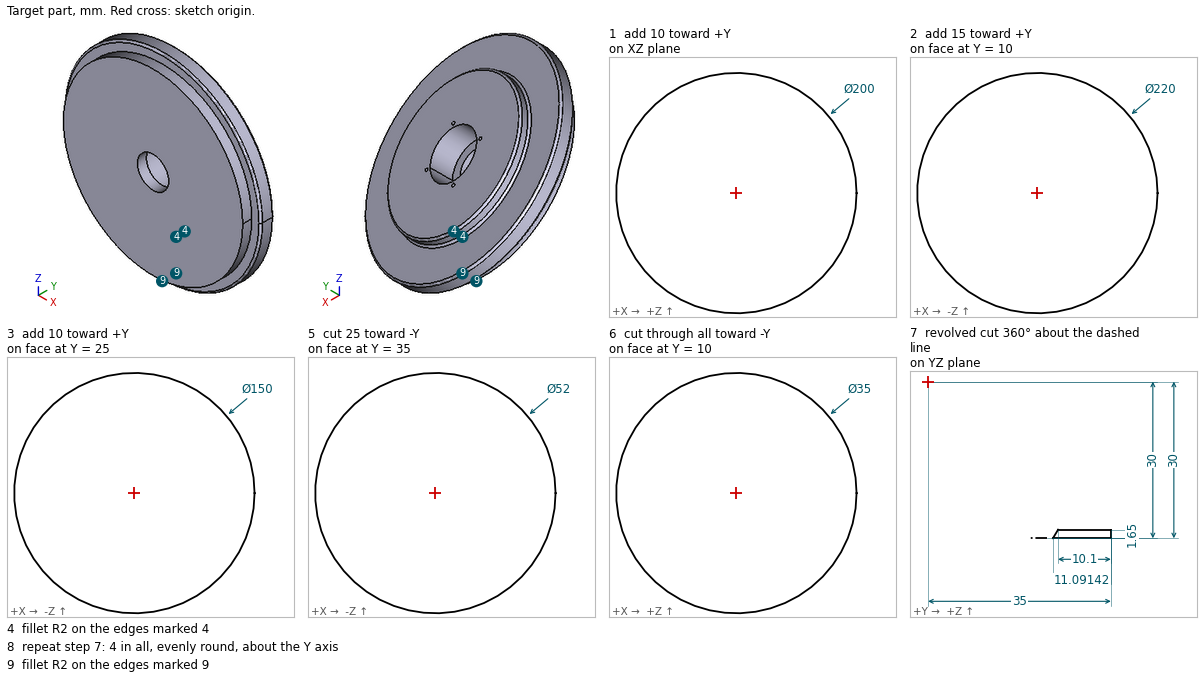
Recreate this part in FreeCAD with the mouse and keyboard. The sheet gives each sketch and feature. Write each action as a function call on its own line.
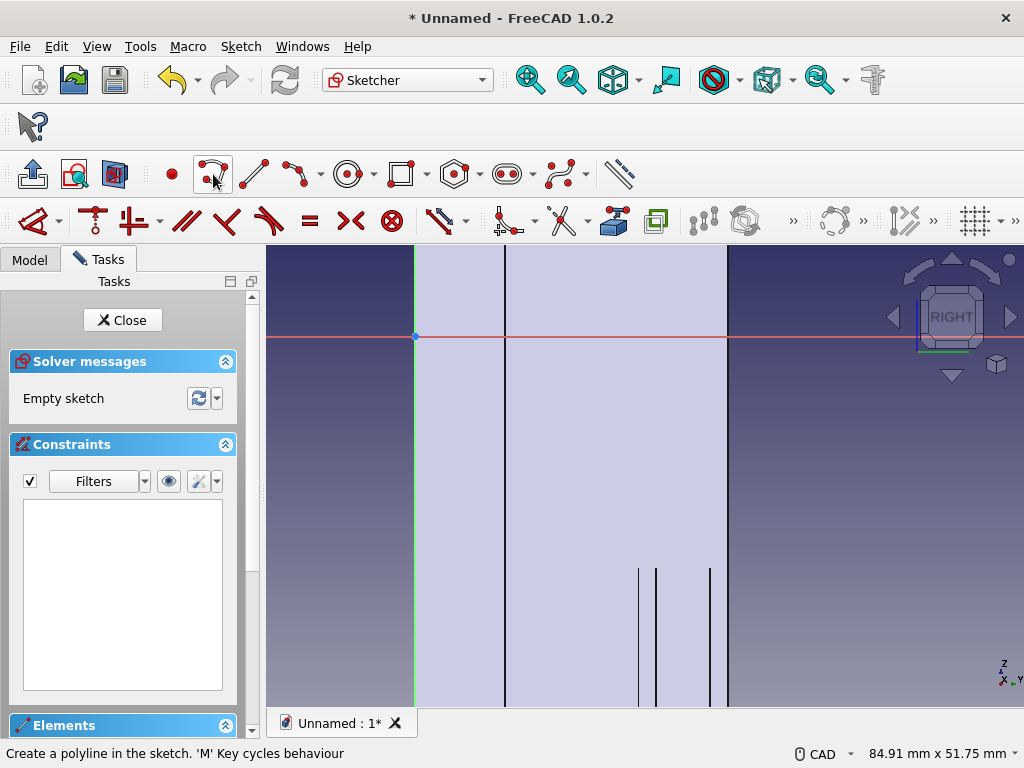
click(638, 590)
click(629, 605)
click(728, 605)
click(728, 590)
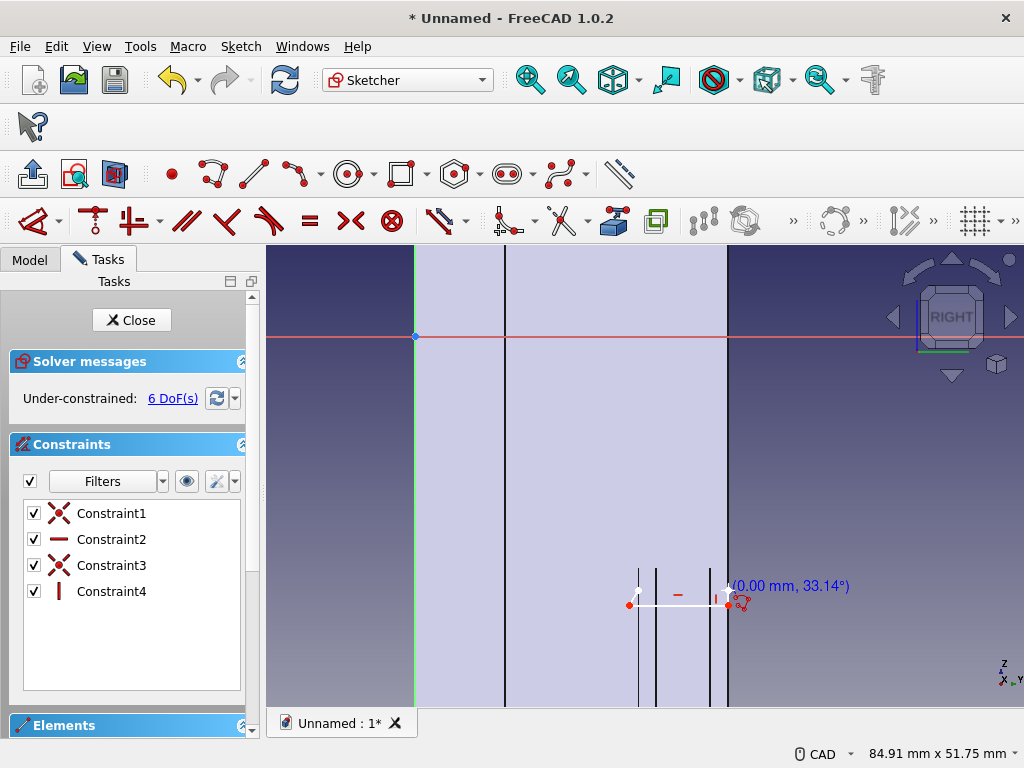
scroll(638, 590, up, 4)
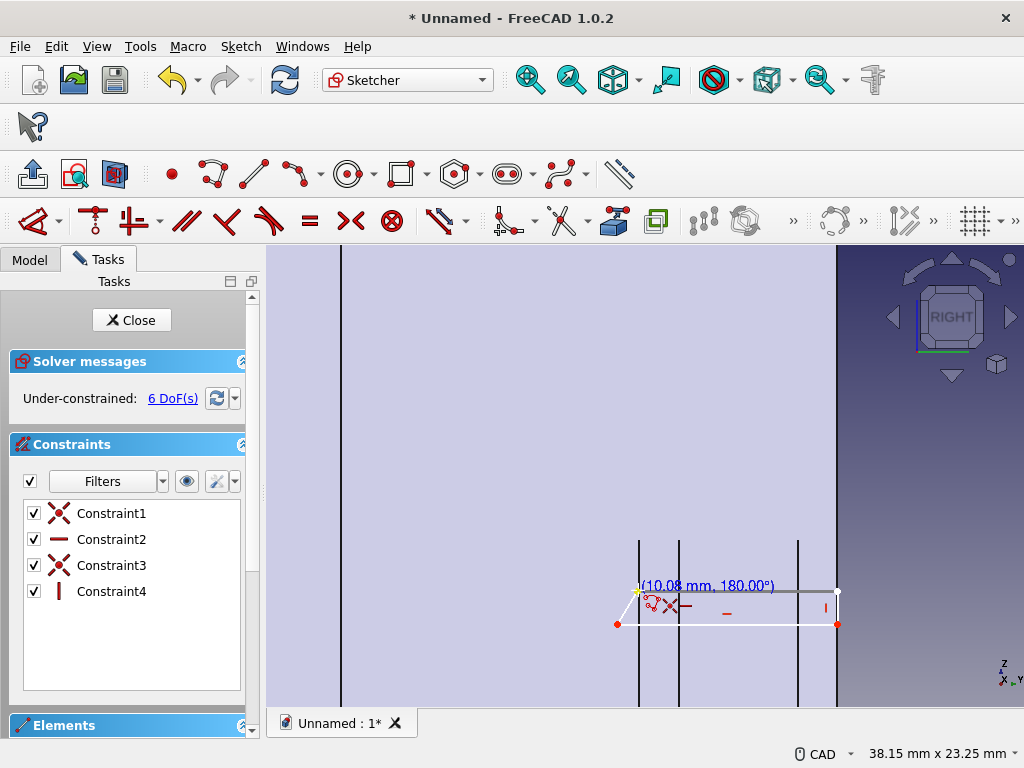
click(637, 591)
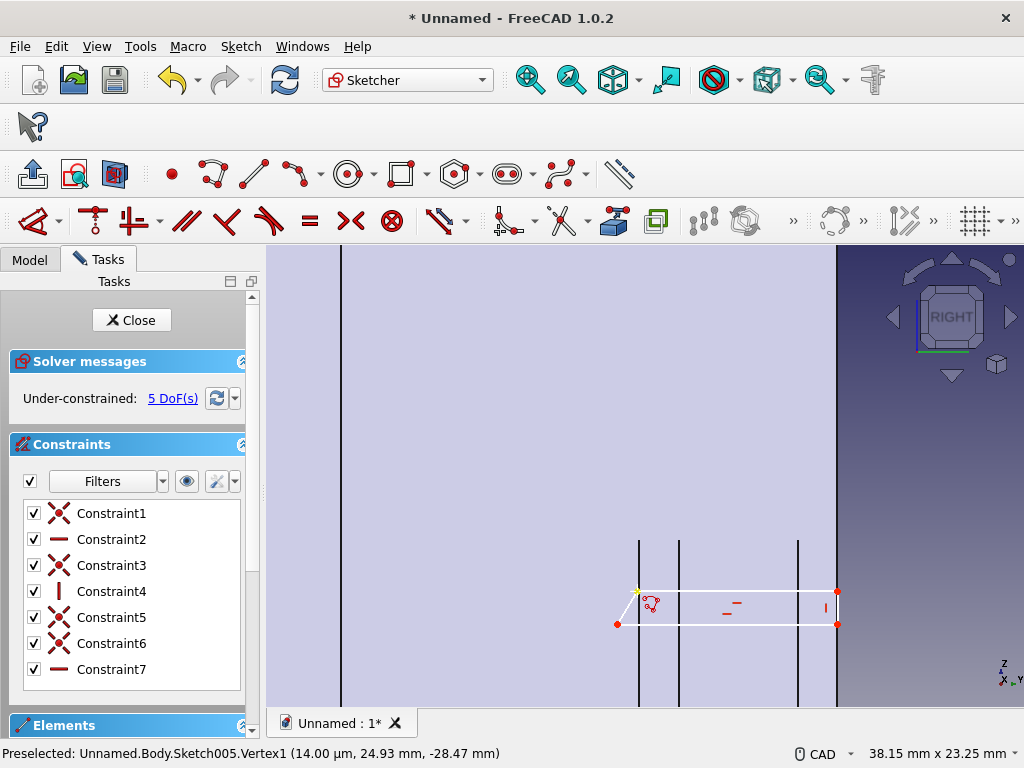
click(254, 174)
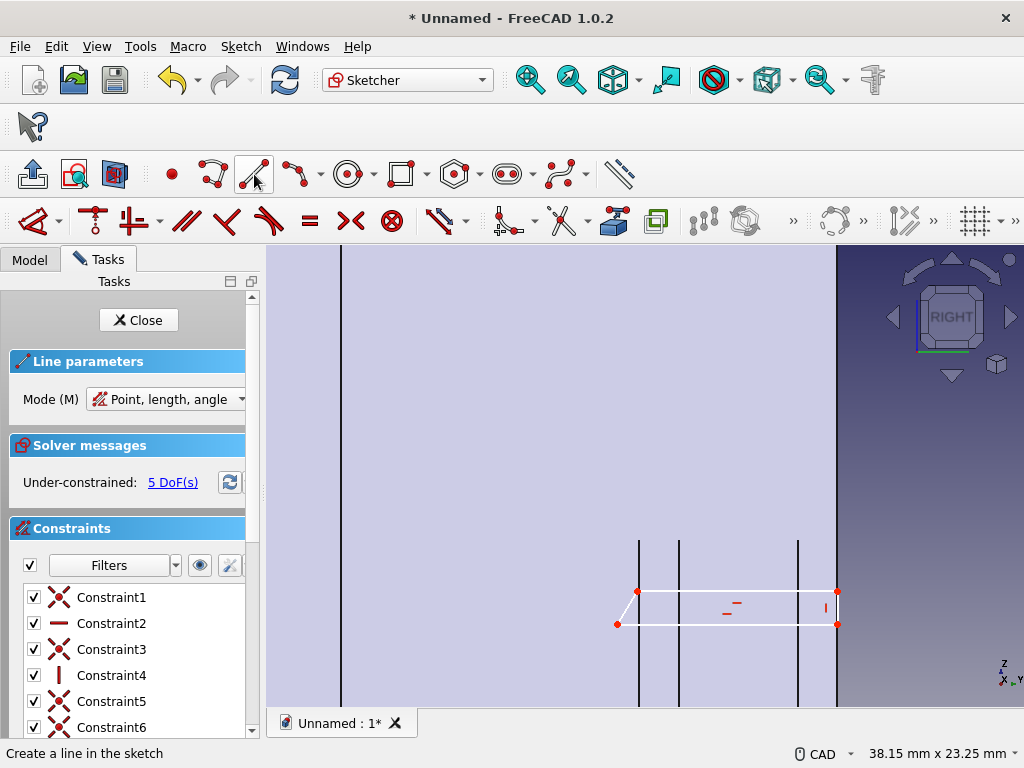
click(595, 622)
click(529, 622)
key(Escape)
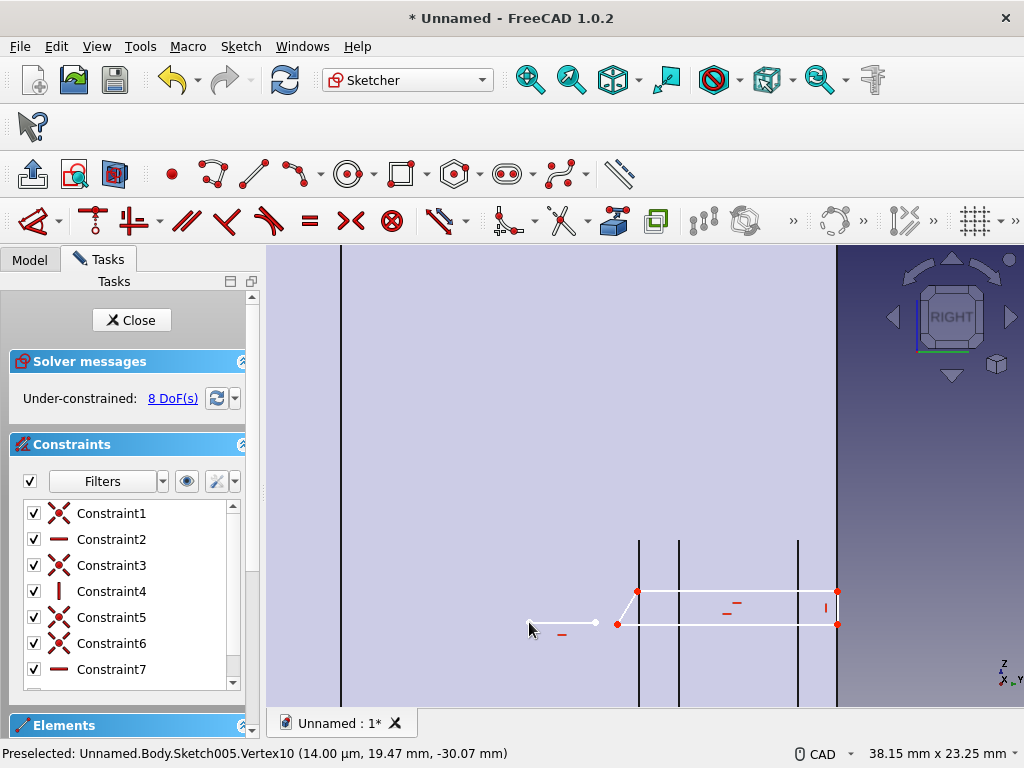
click(575, 623)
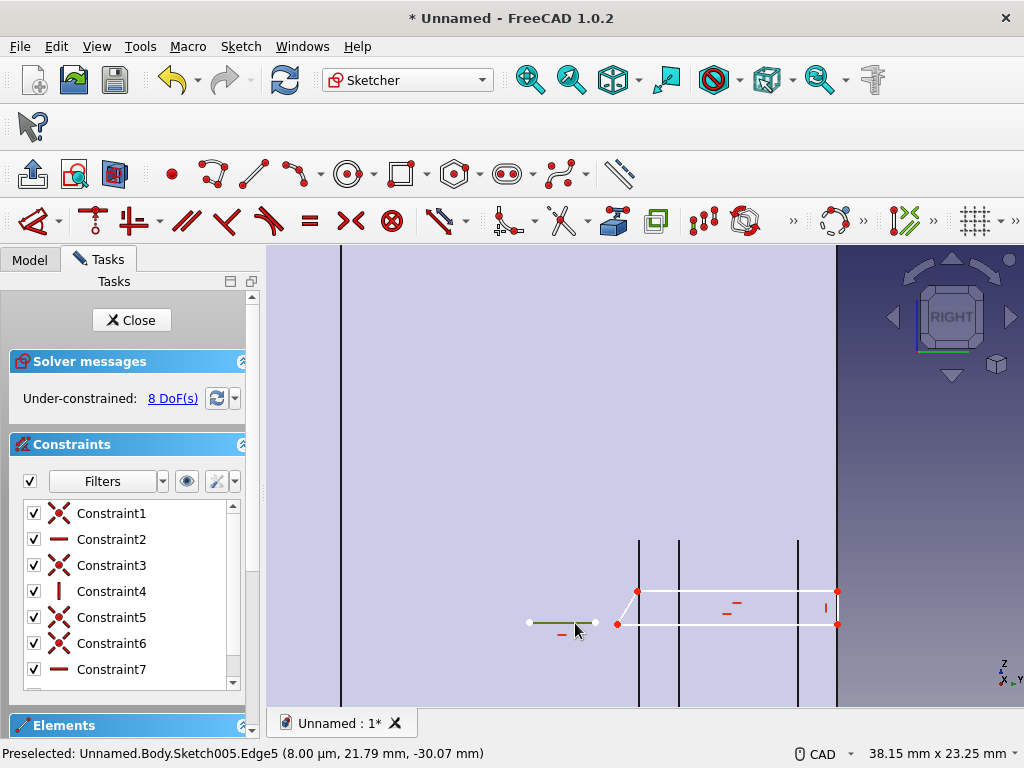
click(620, 174)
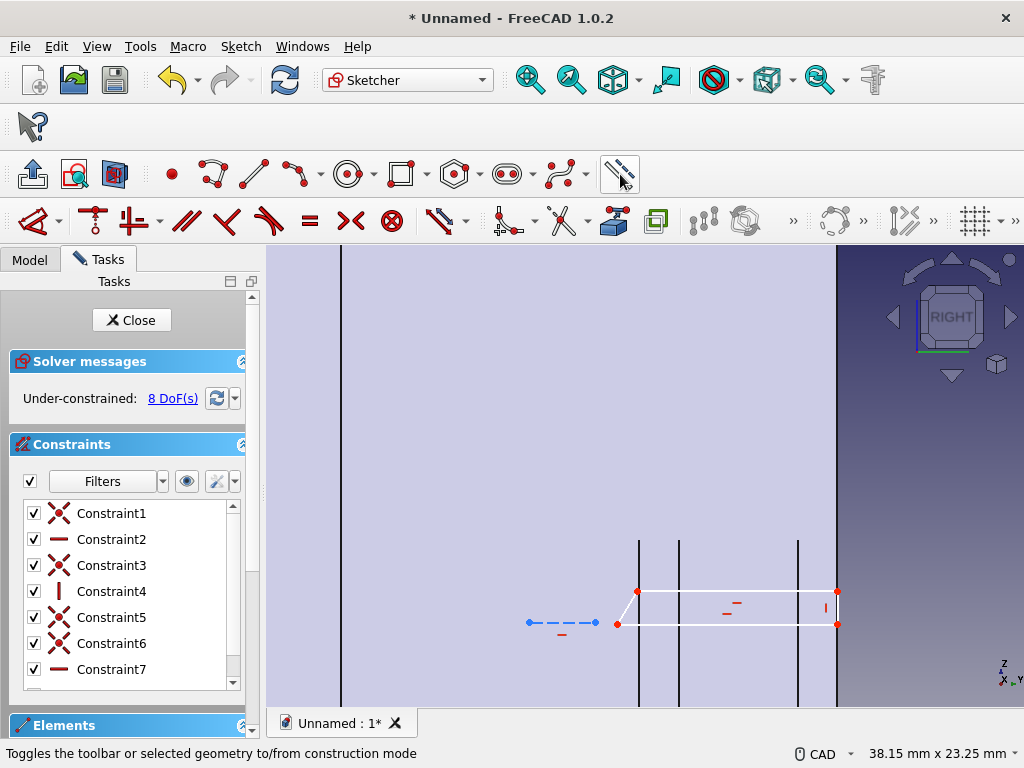
click(32, 222)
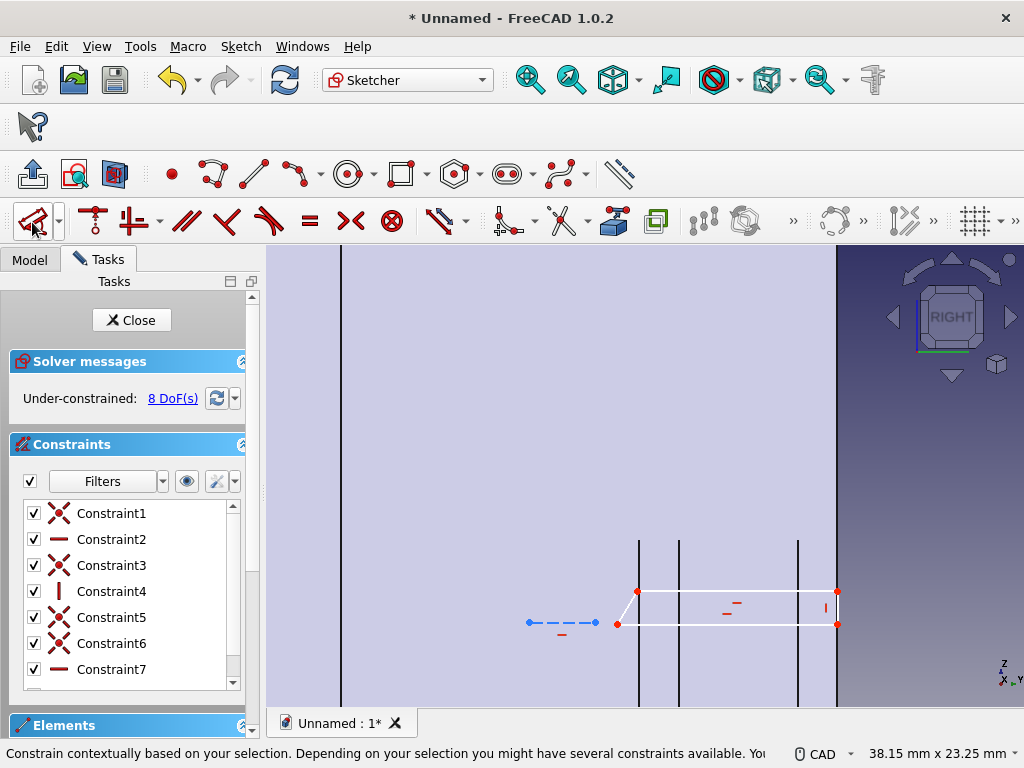
click(617, 625)
click(651, 449)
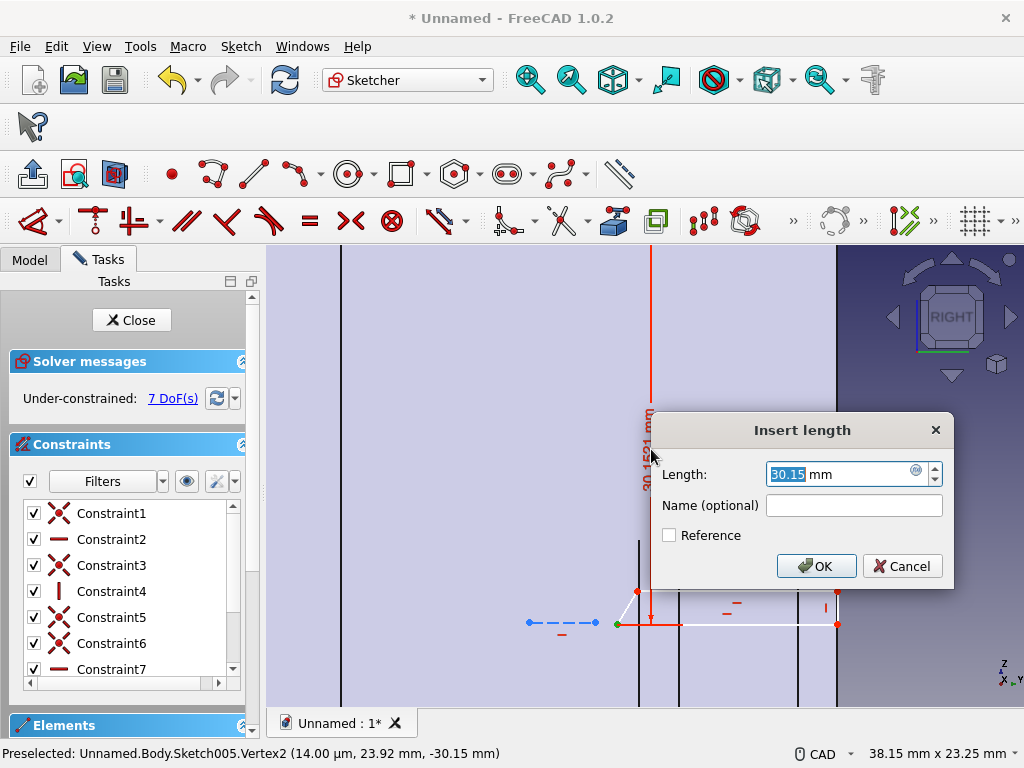
text(30)
key(Return)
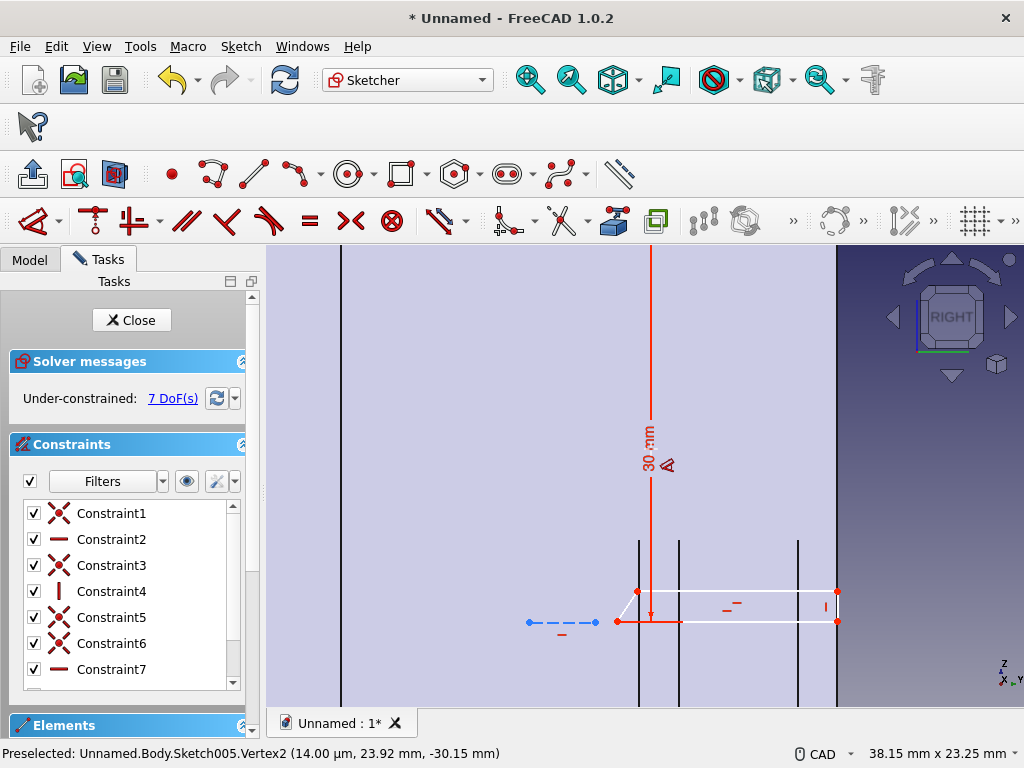
click(838, 622)
click(566, 656)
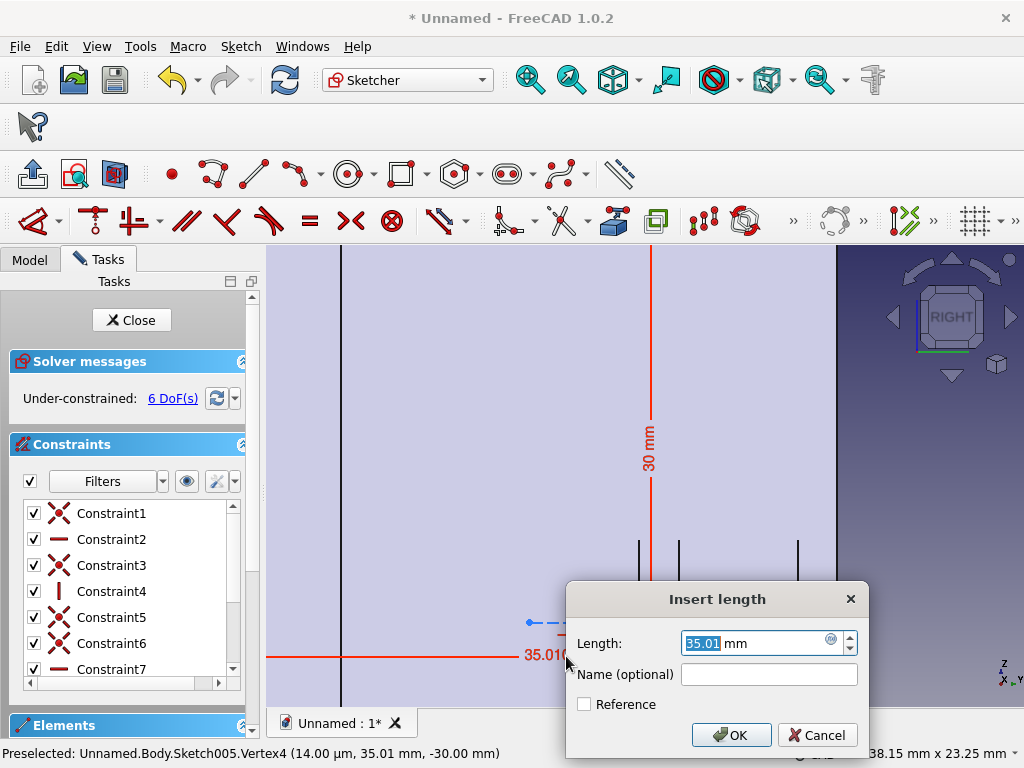
text(35)
key(Return)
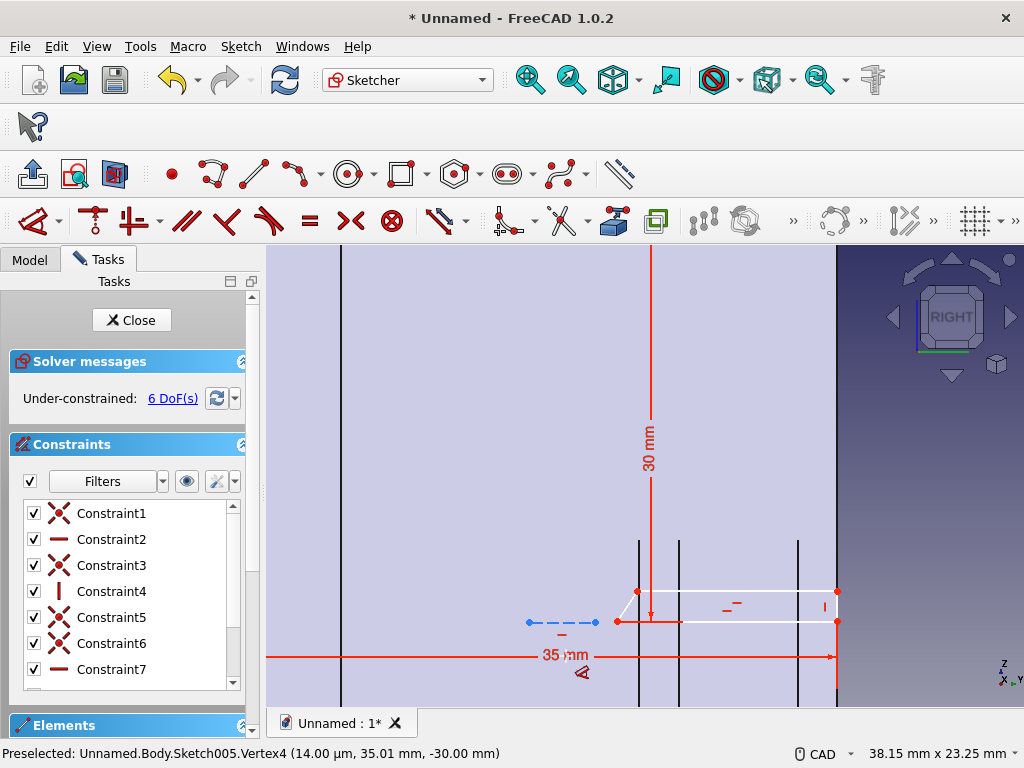
click(595, 623)
click(629, 368)